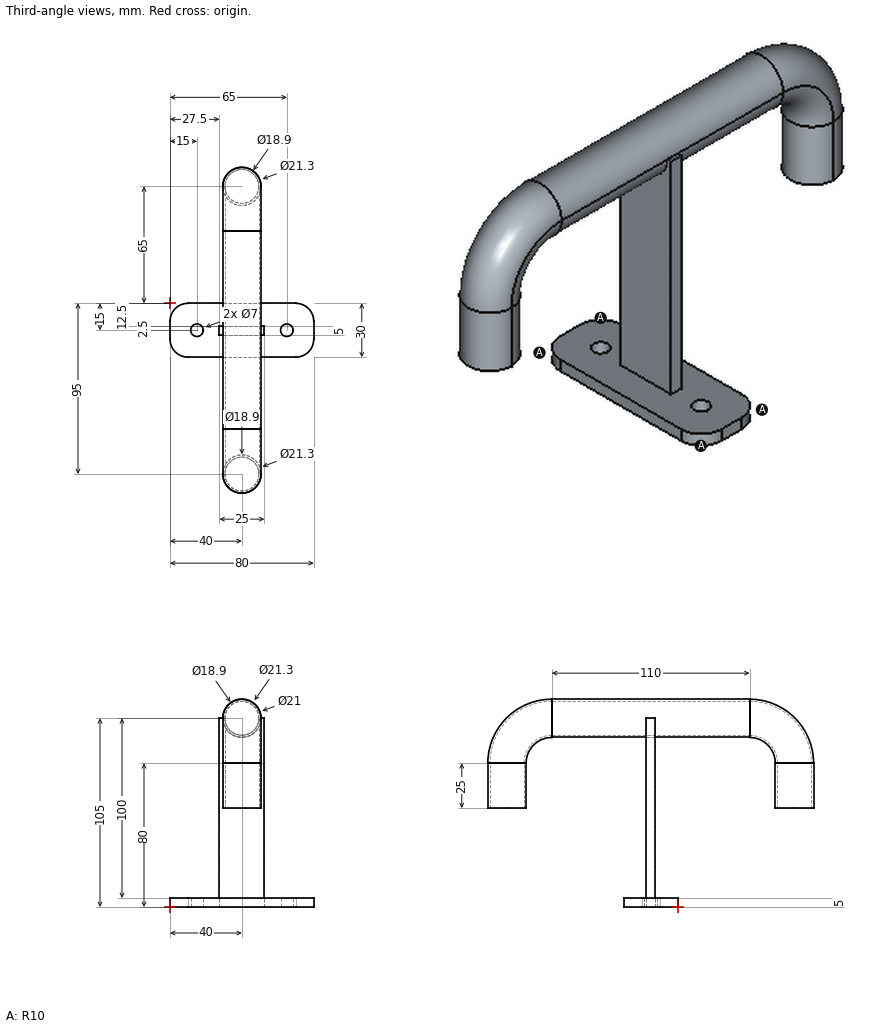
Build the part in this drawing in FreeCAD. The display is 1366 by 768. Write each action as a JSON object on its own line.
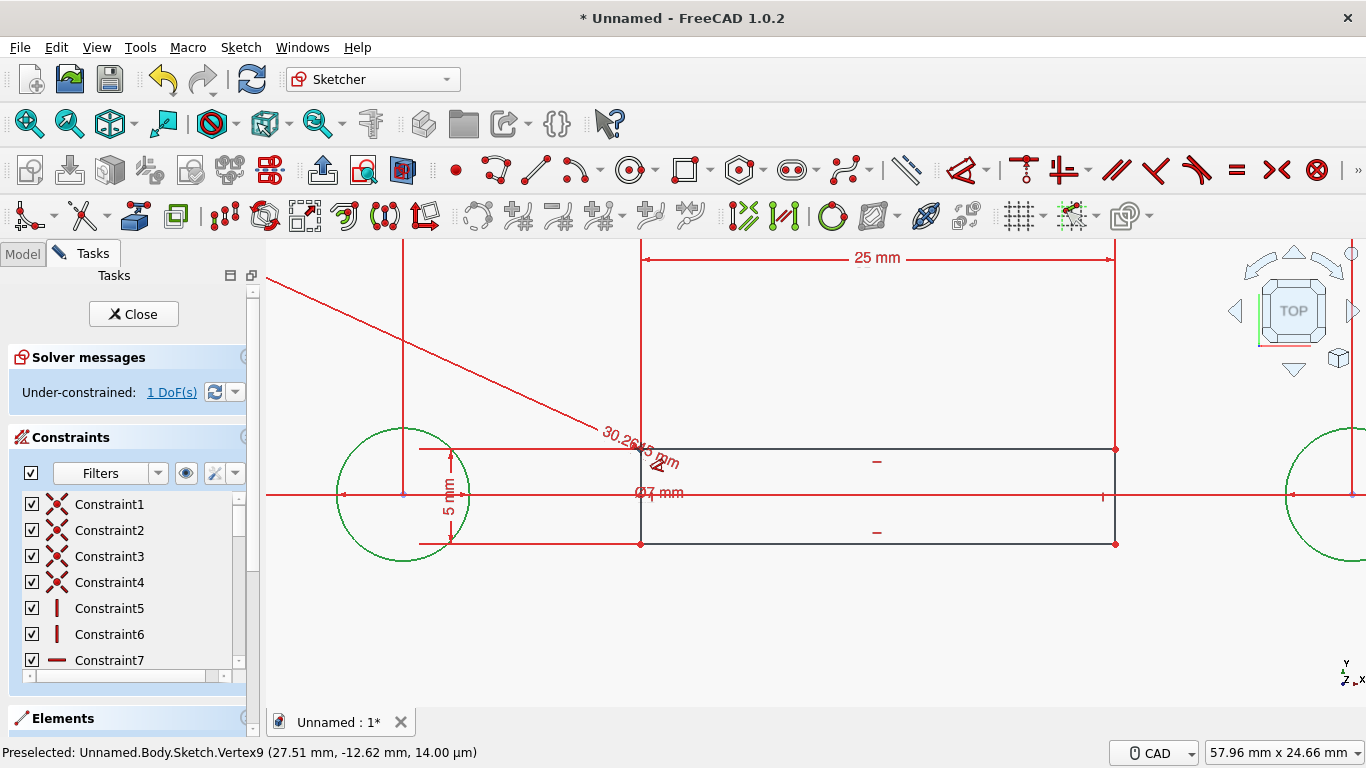
{"action": "left_click", "coordinate": [403, 495]}
{"action": "left_click", "coordinate": [369, 472]}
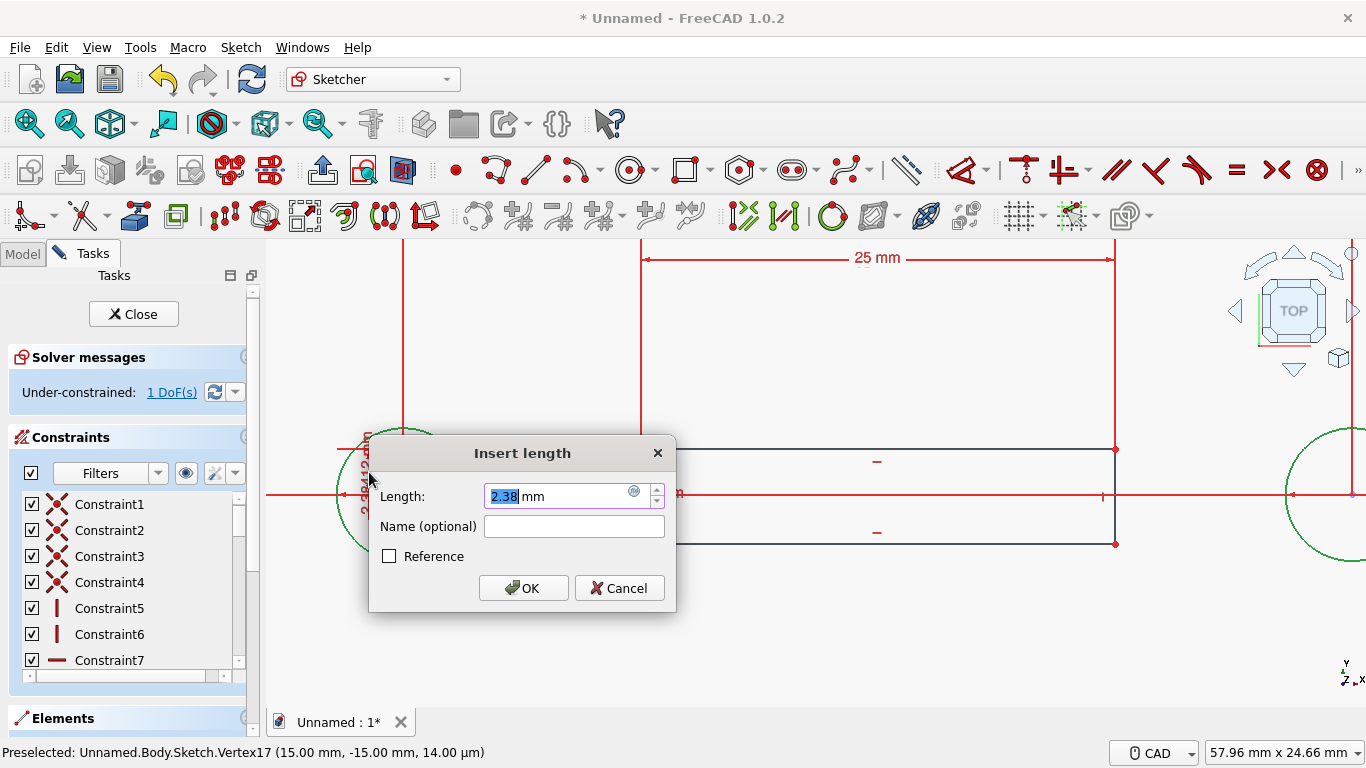
{"action": "type", "text": "2.5"}
{"action": "key", "text": "Return"}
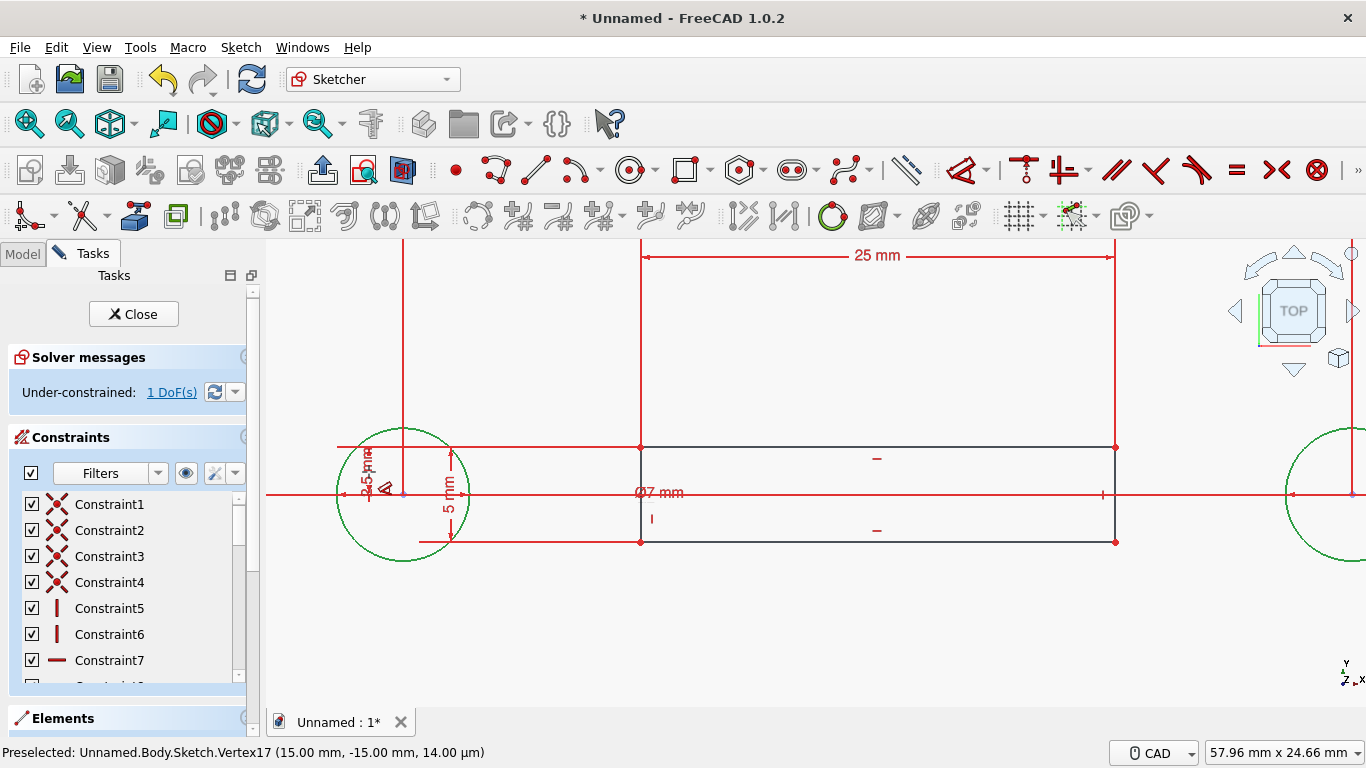
{"action": "left_click", "coordinate": [641, 447]}
{"action": "left_click", "coordinate": [547, 481]}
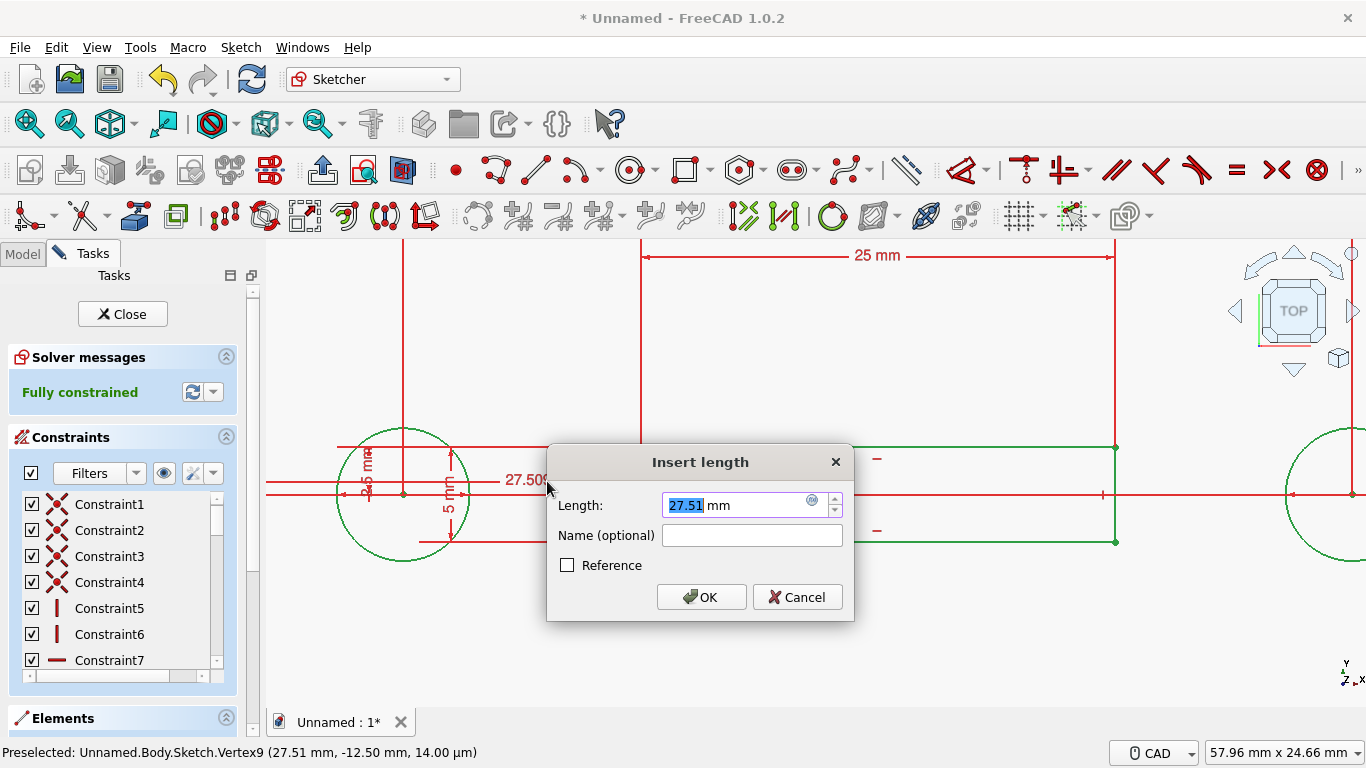
{"action": "type", "text": "27.5"}
{"action": "key", "text": "Return"}
{"action": "key", "text": "Escape"}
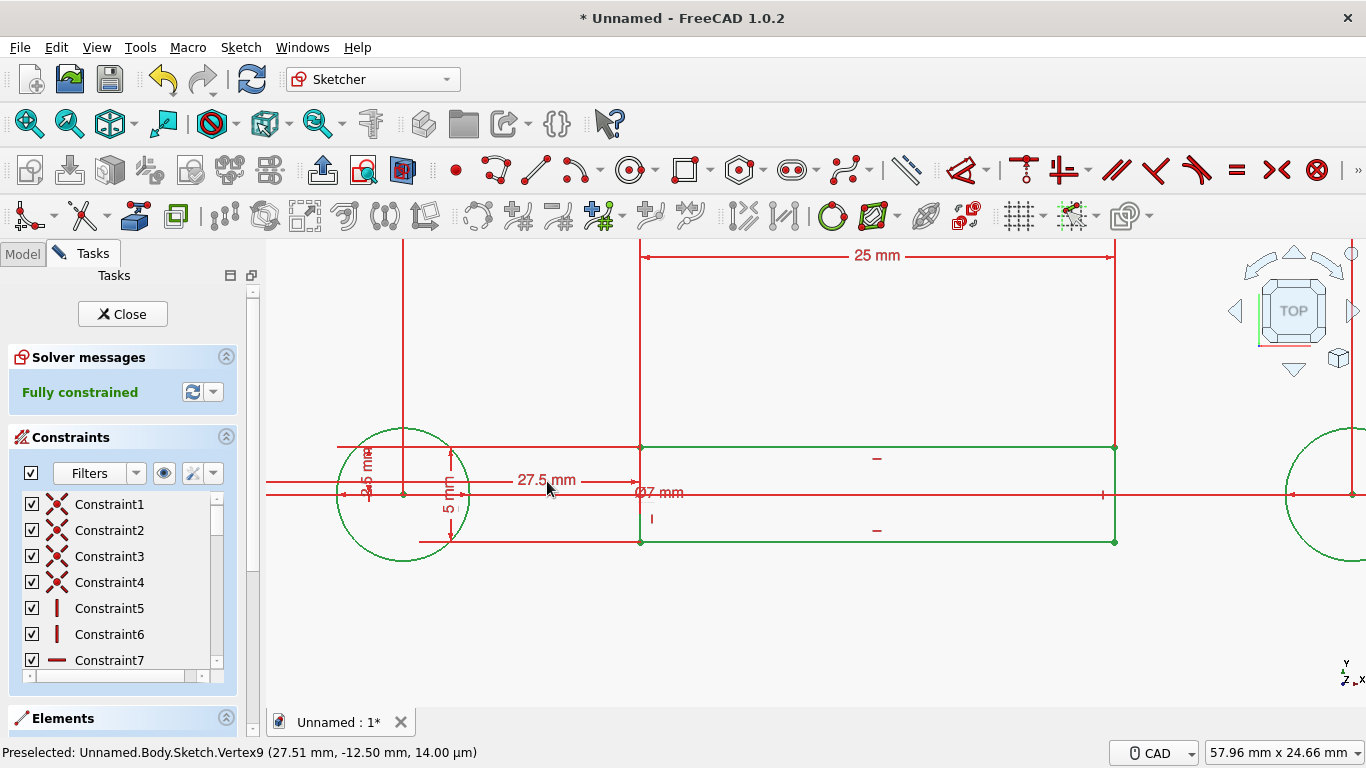
{"action": "left_click", "coordinate": [123, 314]}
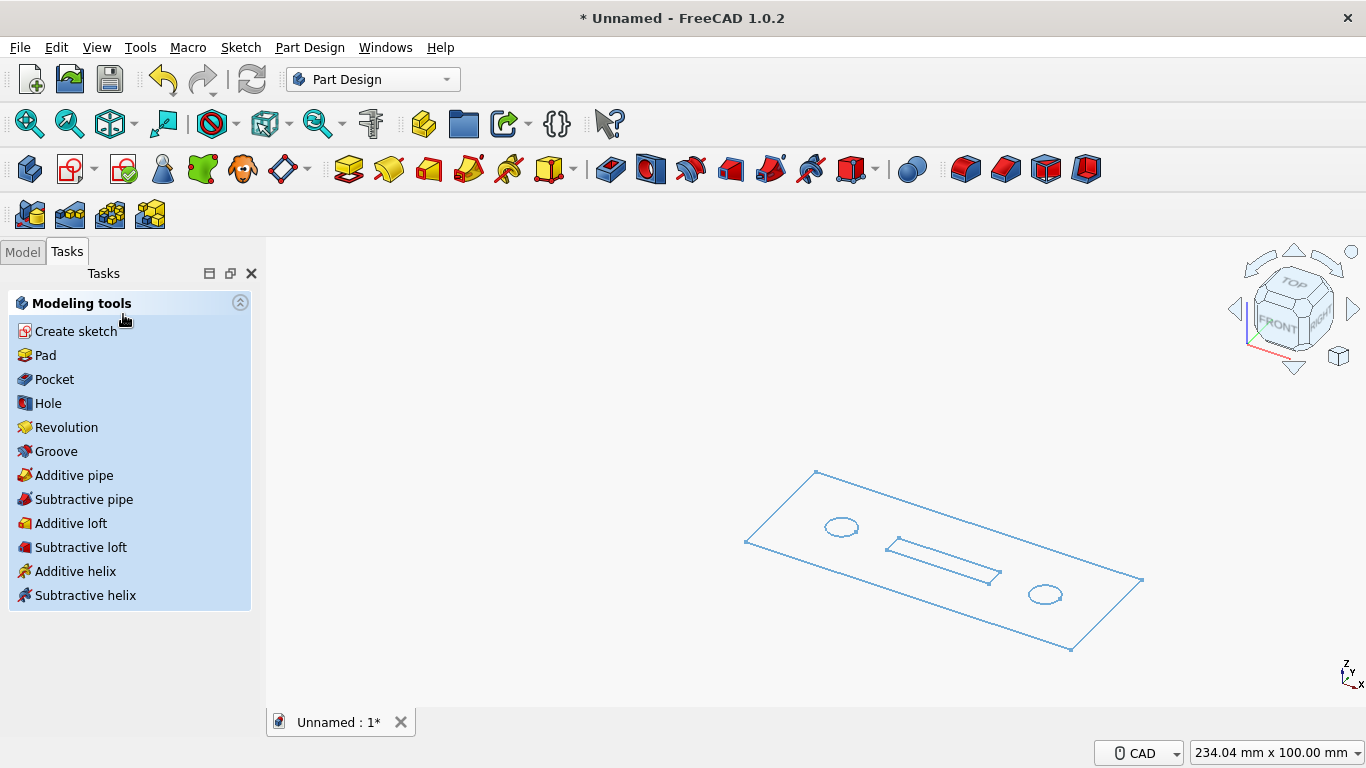
{"action": "left_click", "coordinate": [350, 170]}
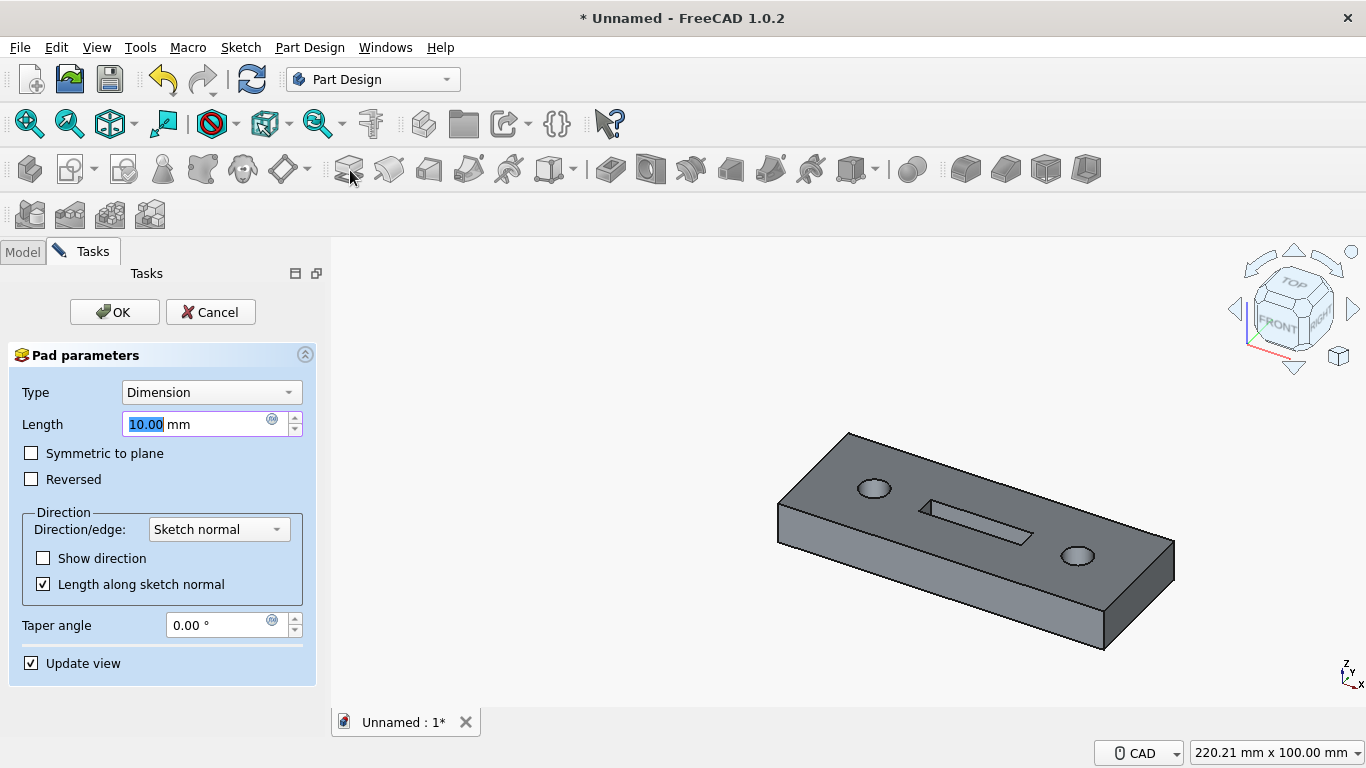
{"action": "type", "text": "5"}
{"action": "key", "text": "Tab"}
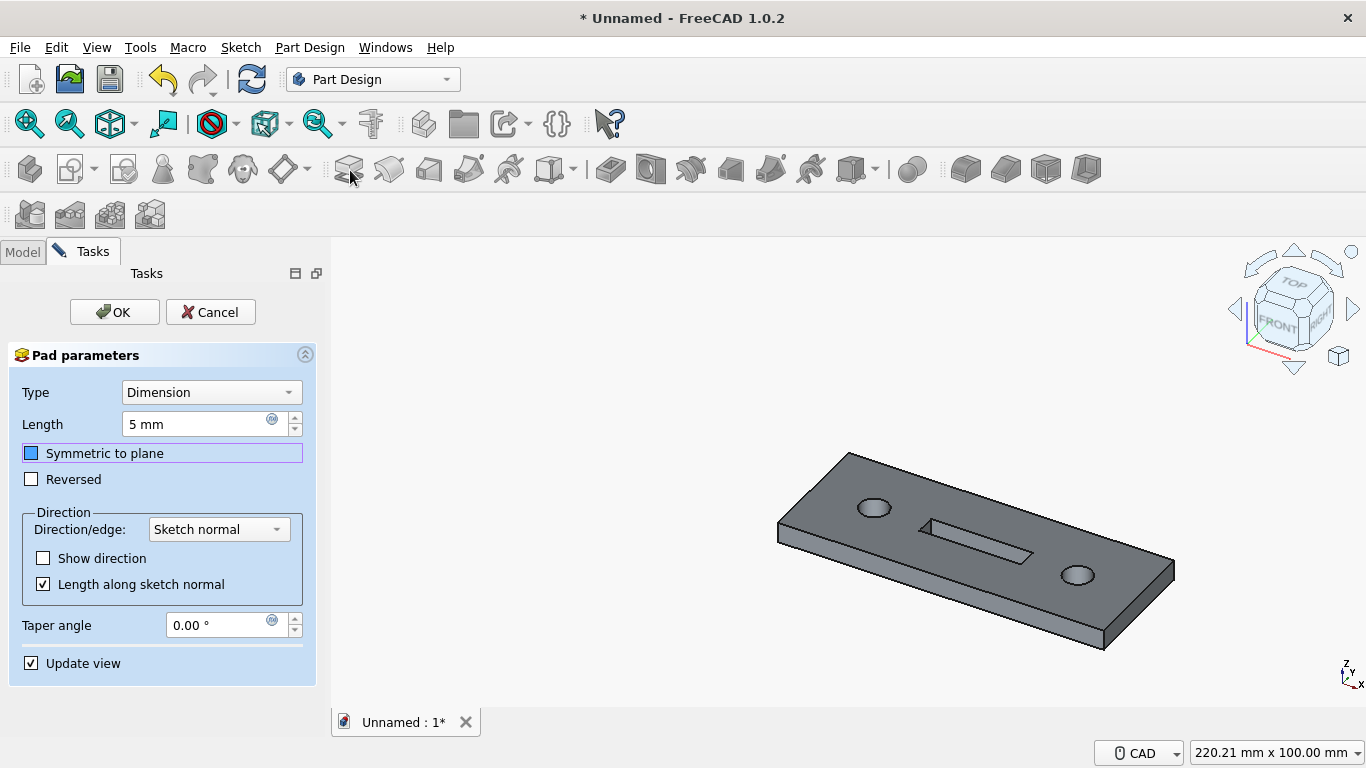
{"action": "left_click", "coordinate": [115, 312]}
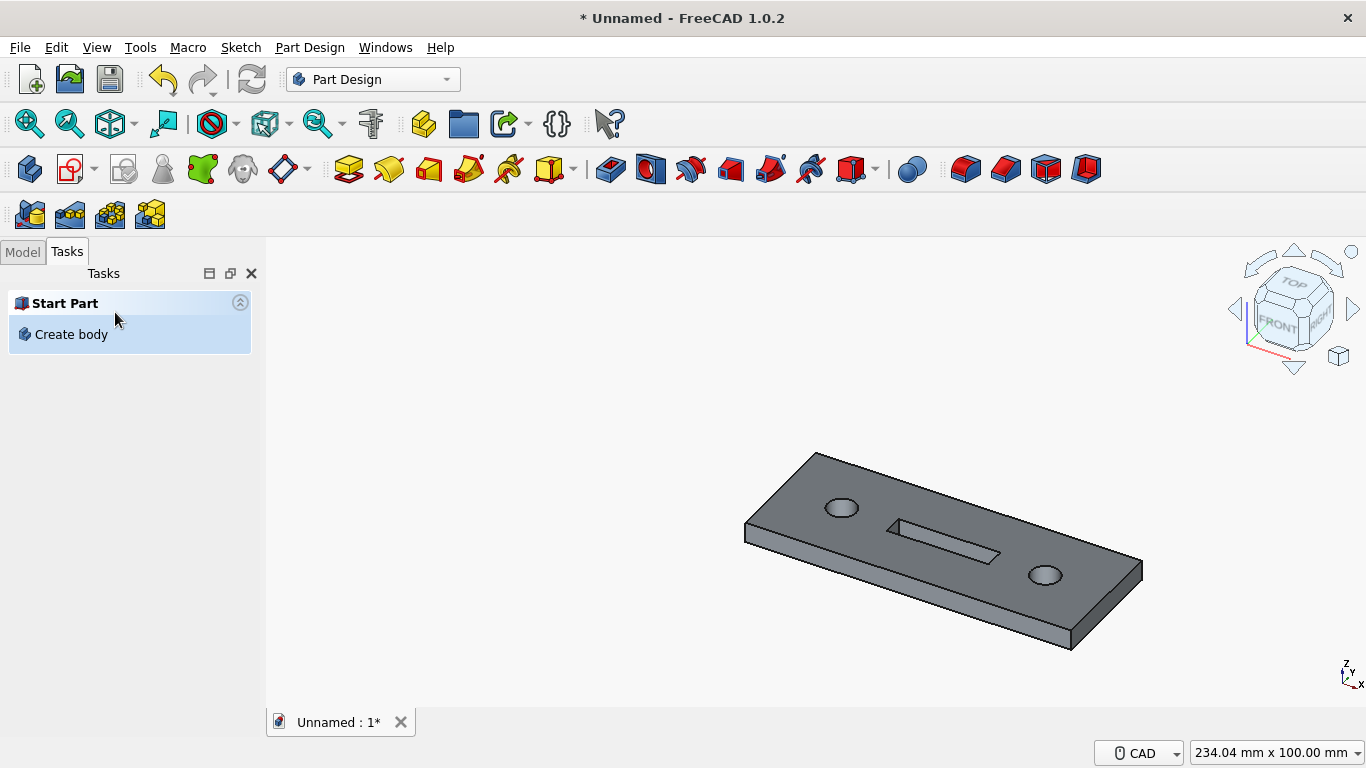
{"action": "left_click", "coordinate": [30, 124]}